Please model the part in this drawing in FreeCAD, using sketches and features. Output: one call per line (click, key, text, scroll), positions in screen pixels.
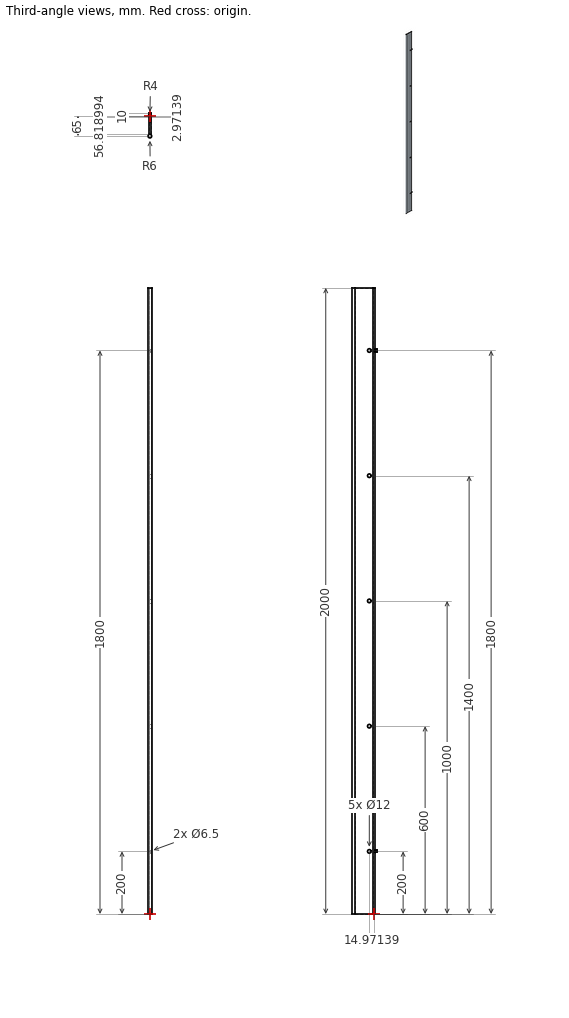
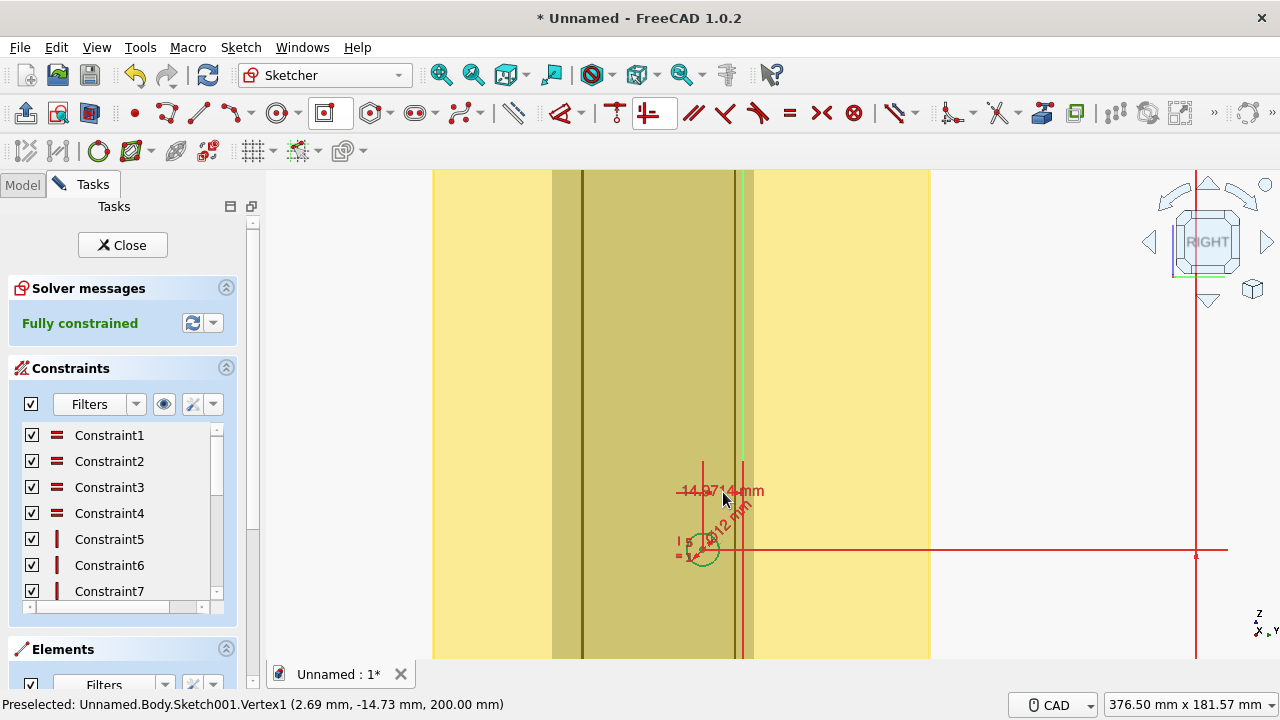
click(123, 245)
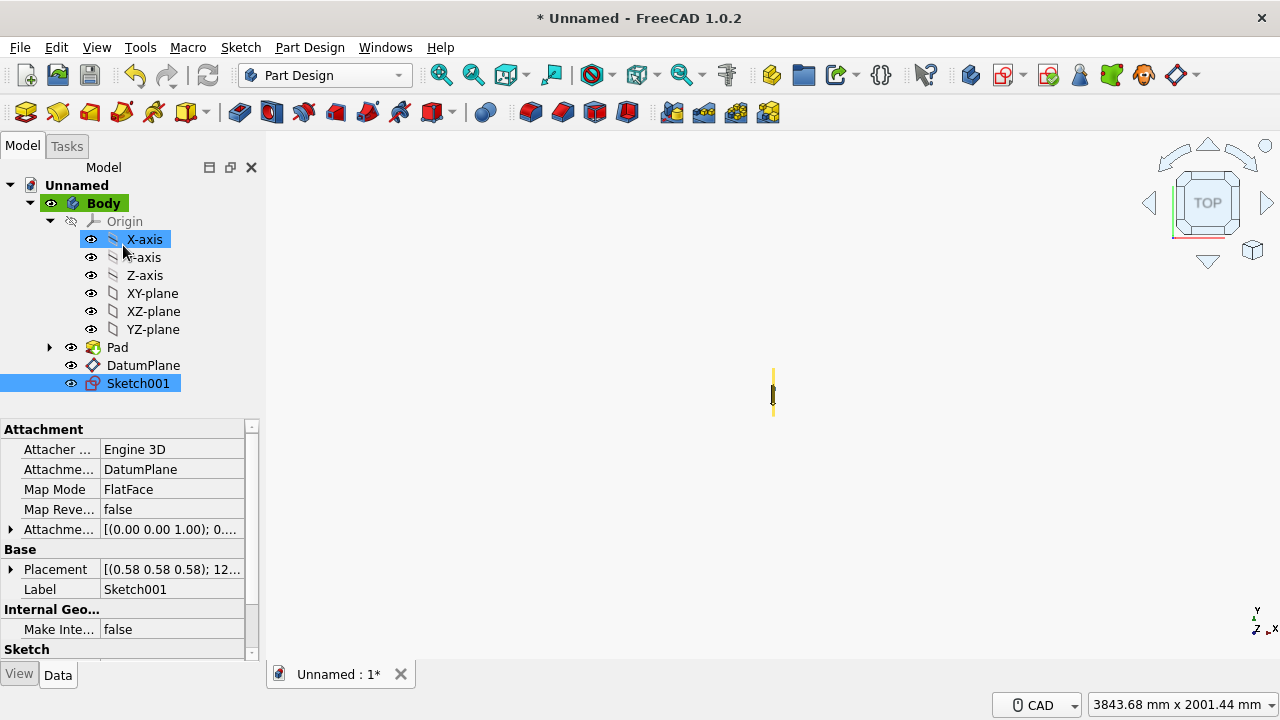
click(240, 112)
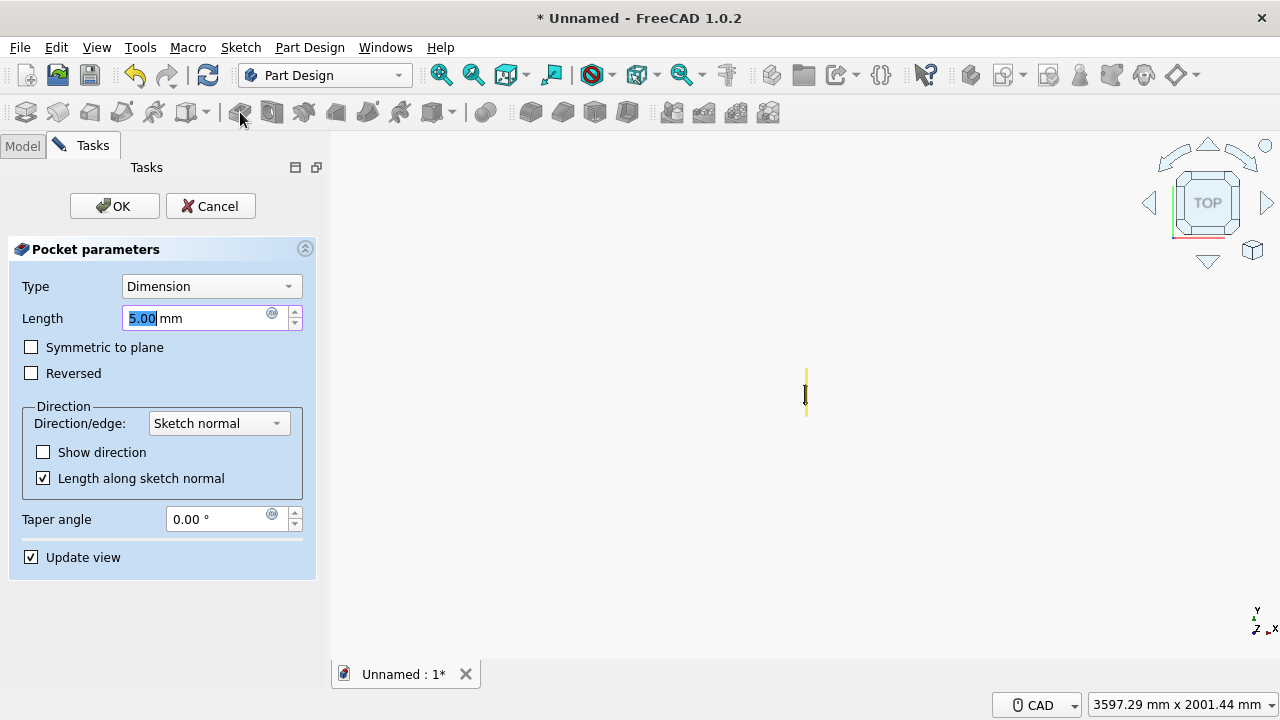
click(212, 286)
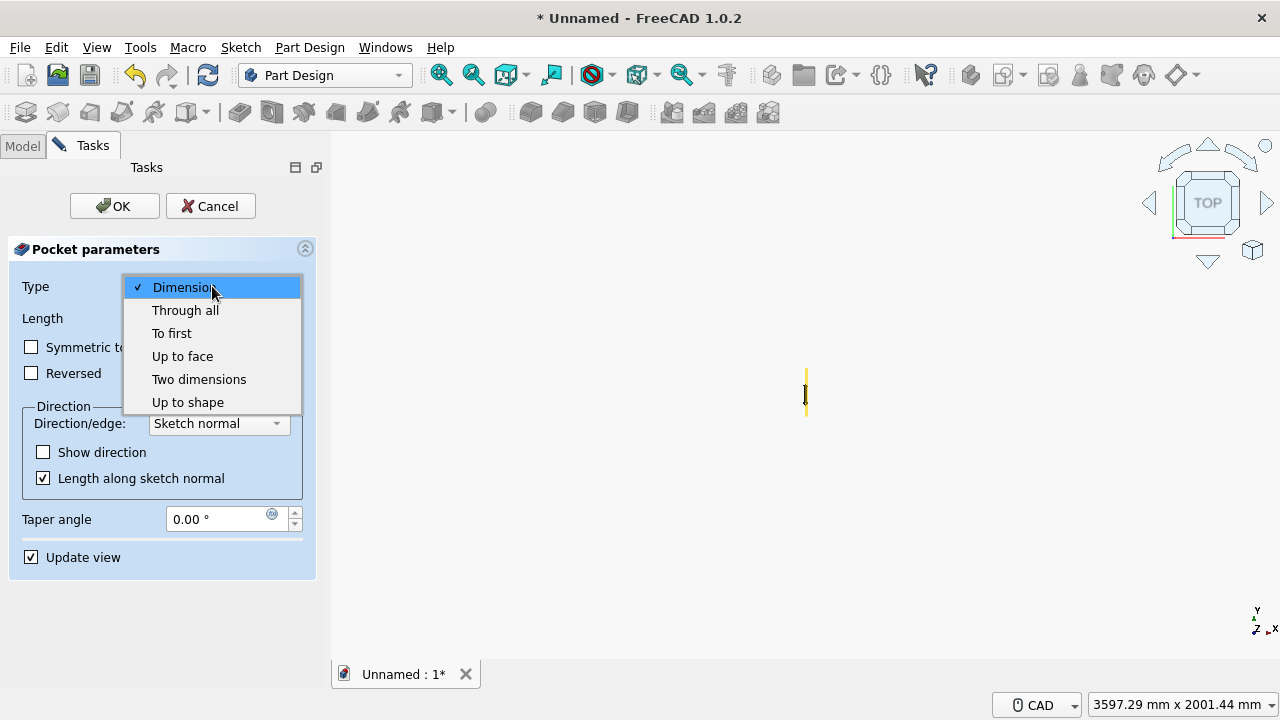
click(212, 310)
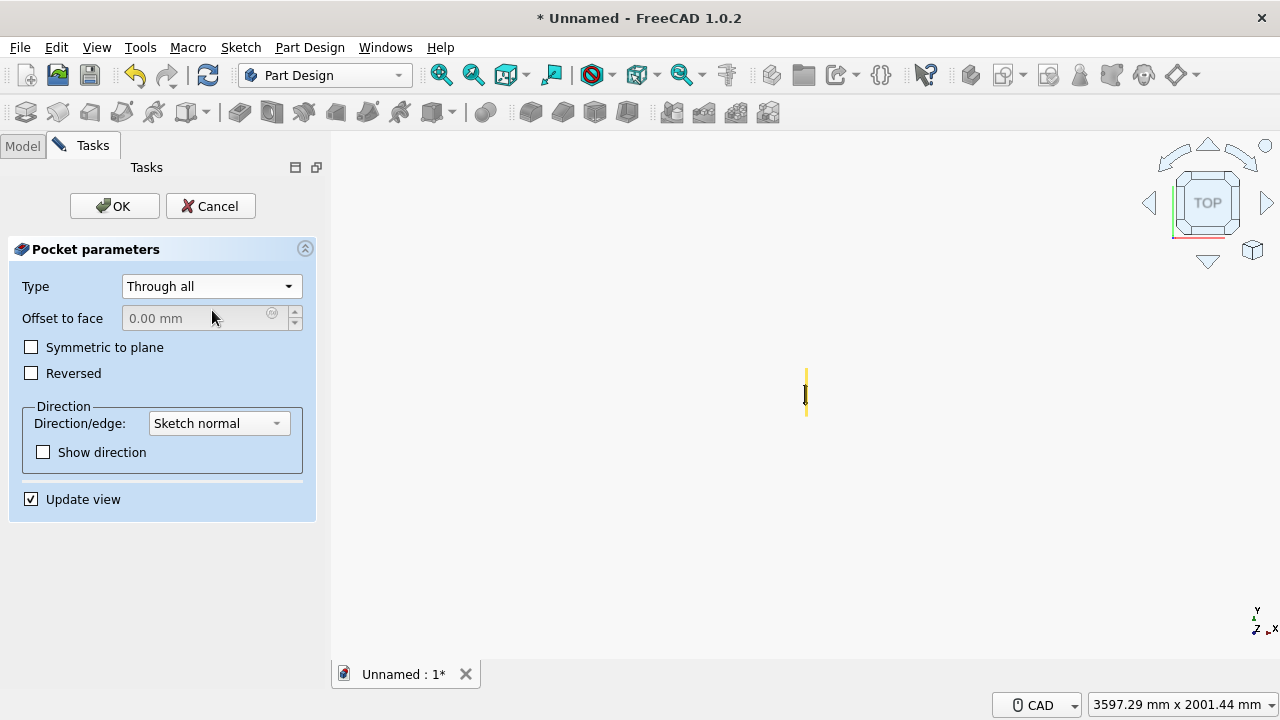
click(115, 206)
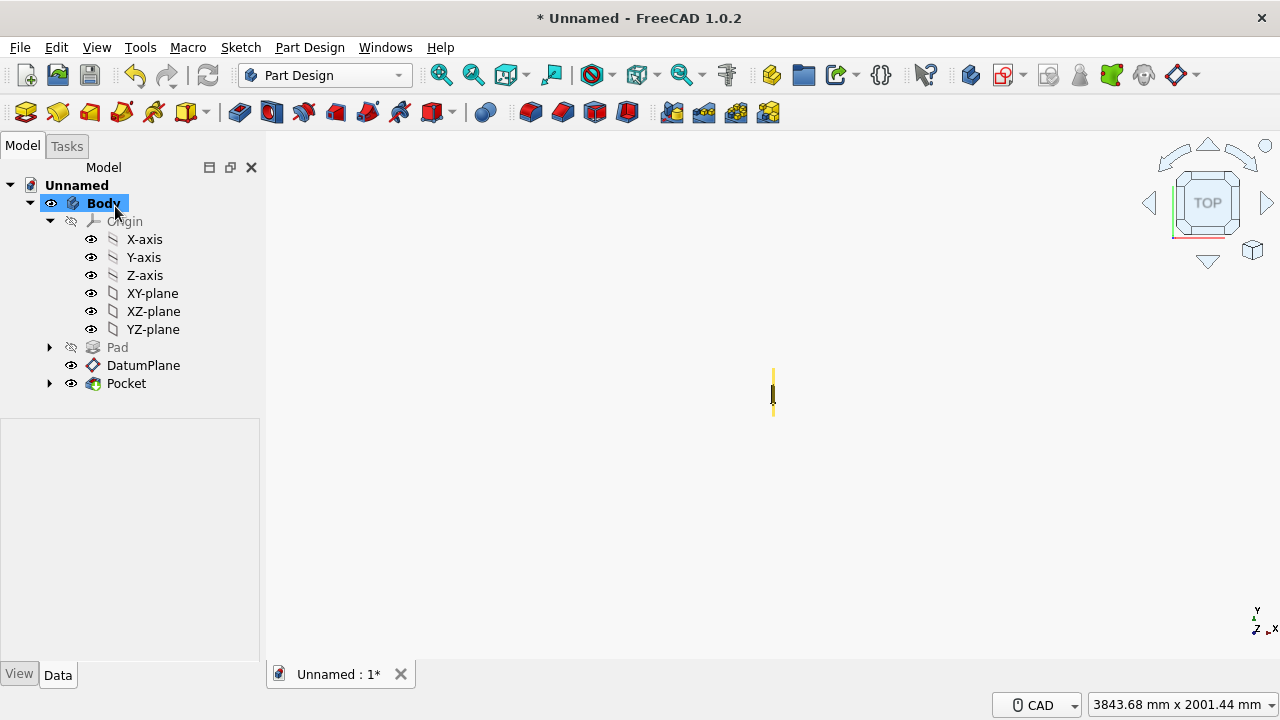
click(116, 365)
key(space)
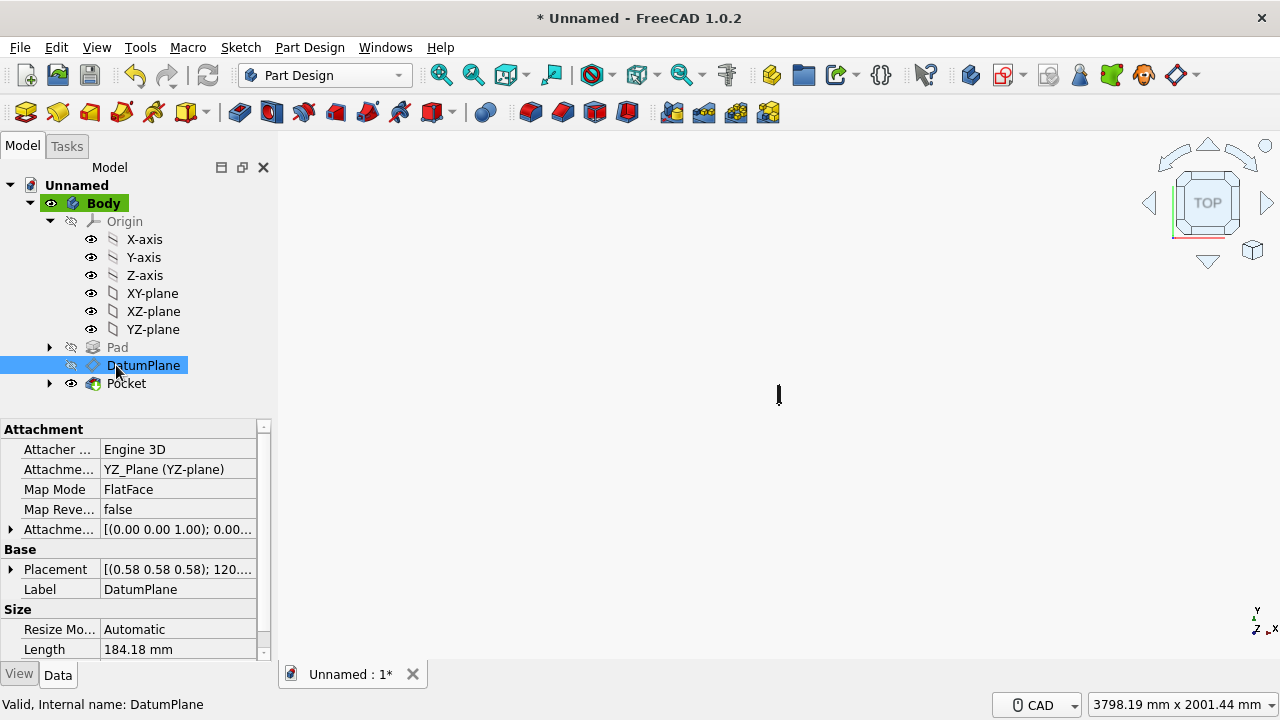
click(442, 76)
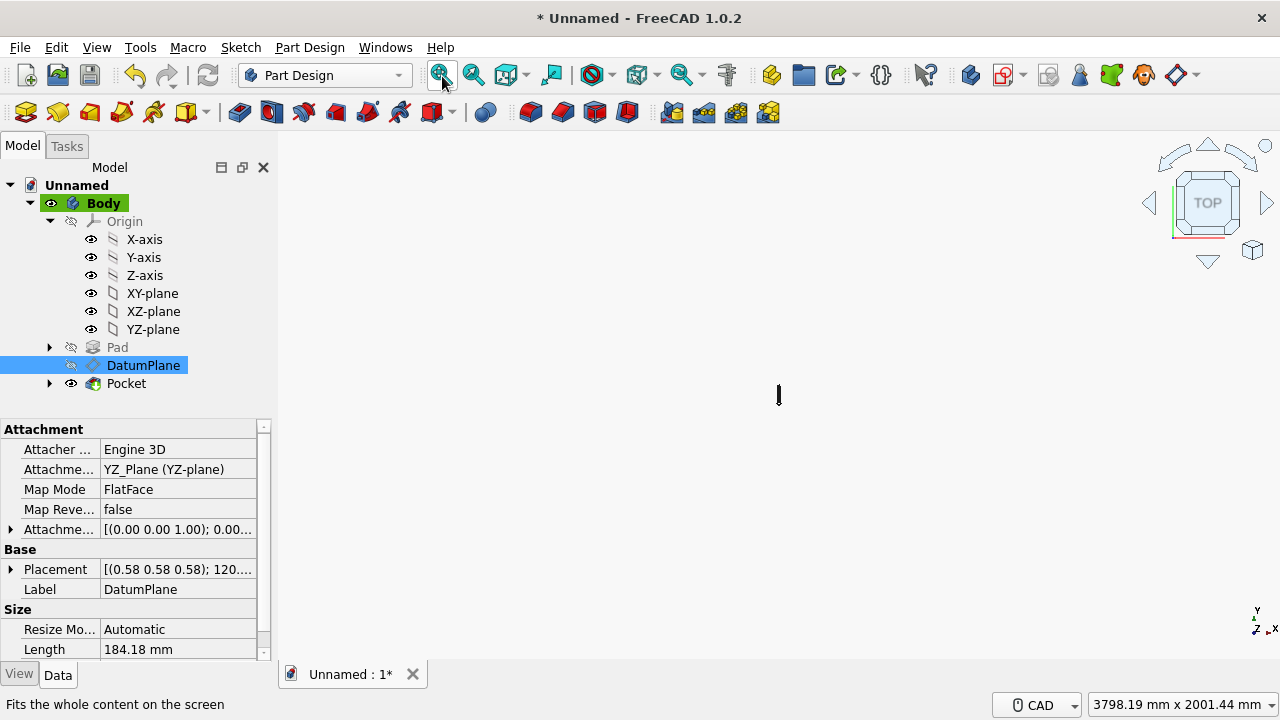
click(318, 619)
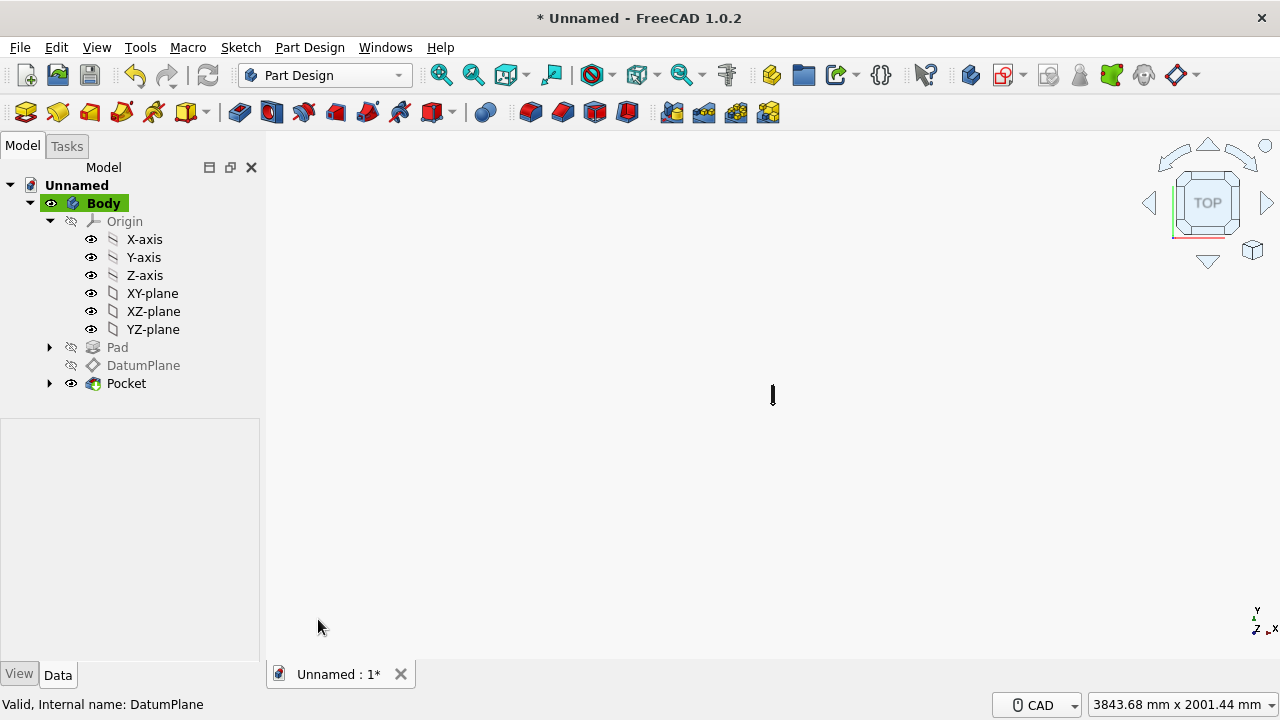
click(1004, 76)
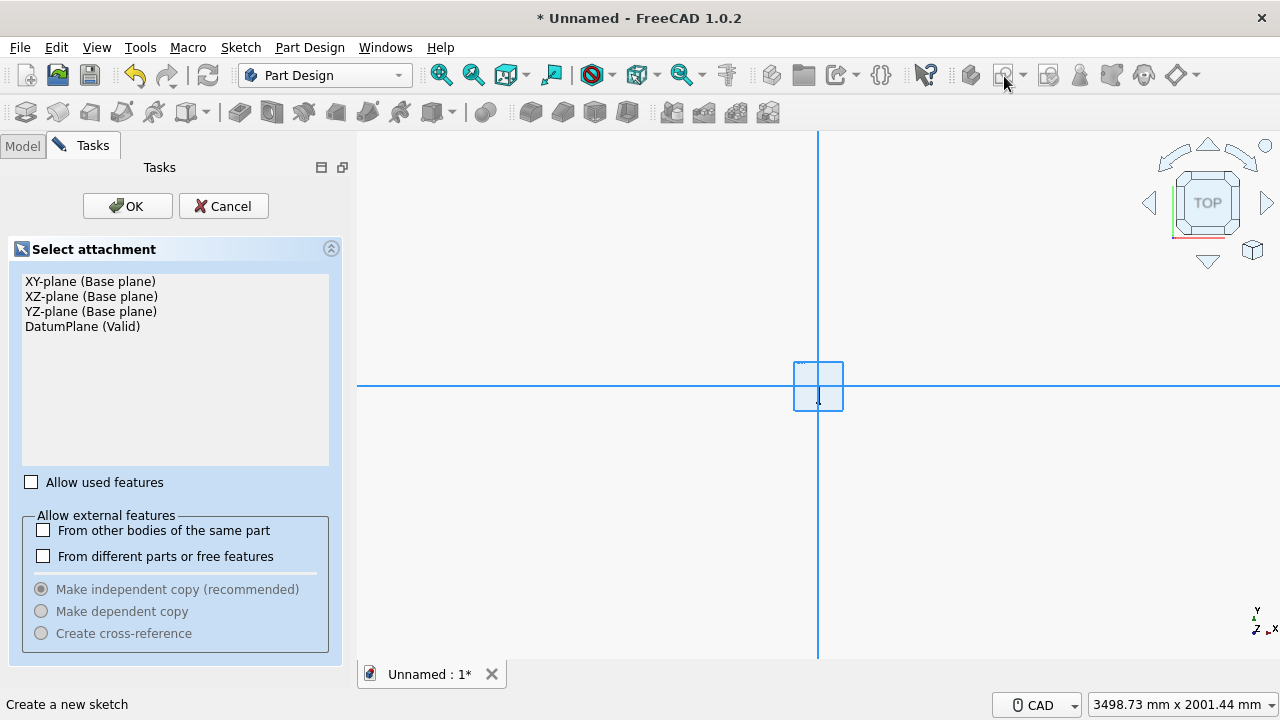
click(82, 296)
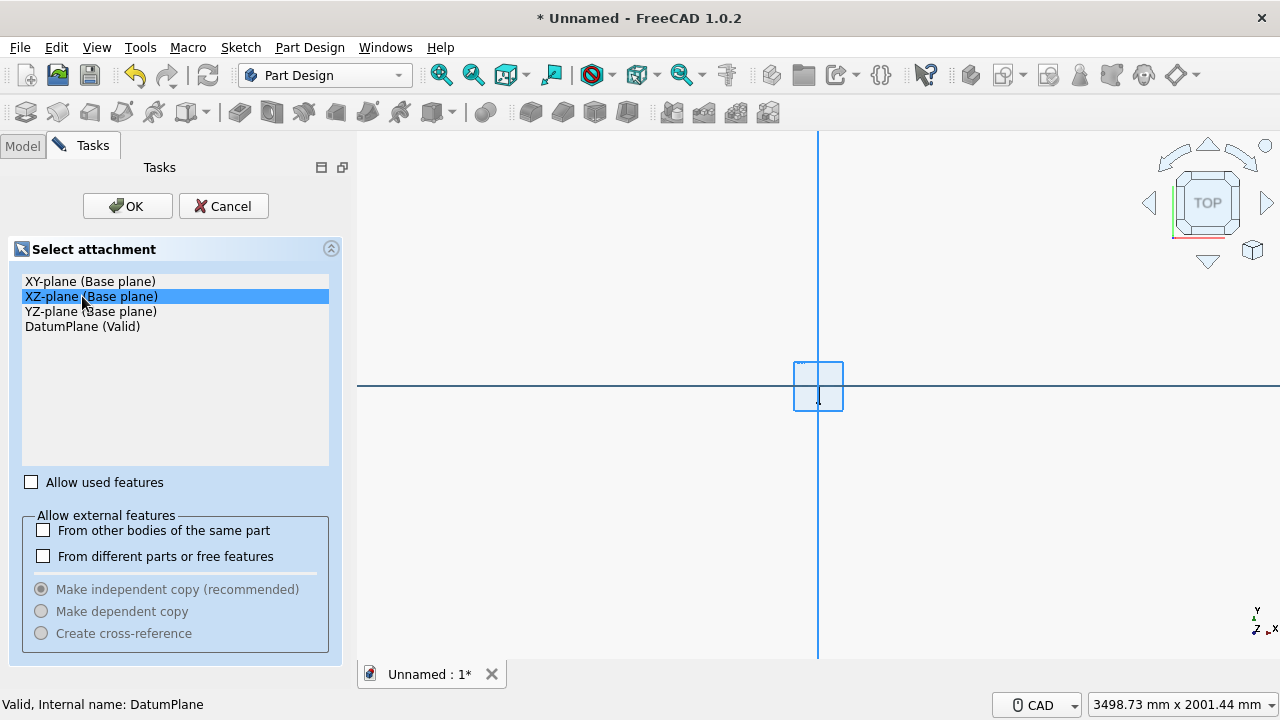
click(128, 206)